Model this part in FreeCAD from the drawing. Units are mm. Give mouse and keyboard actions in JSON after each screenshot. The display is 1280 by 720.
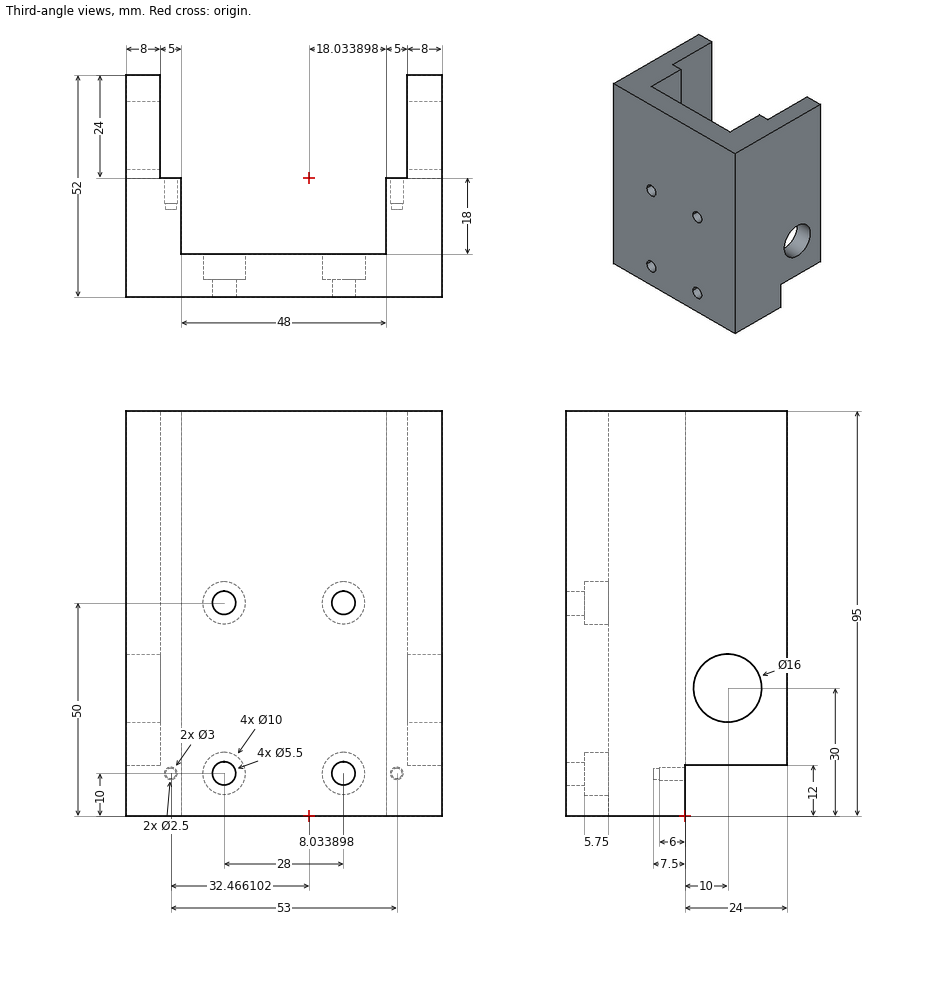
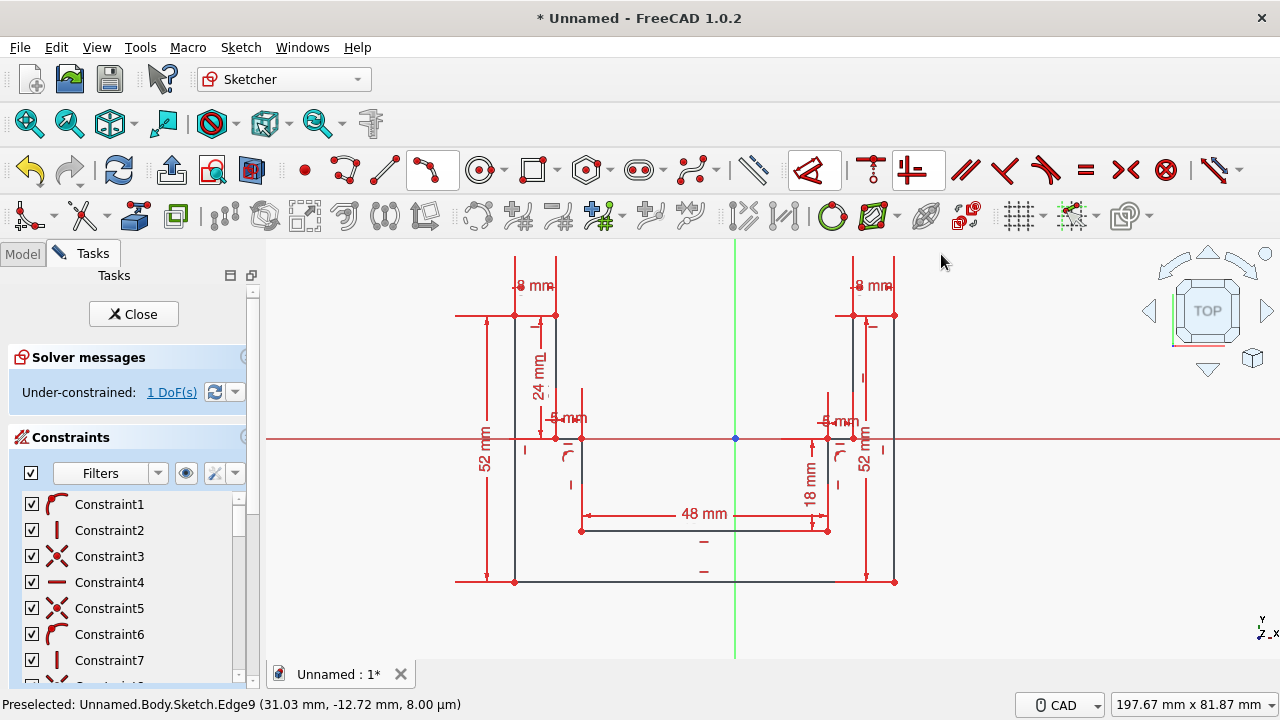
{"action": "left_click", "coordinate": [828, 439]}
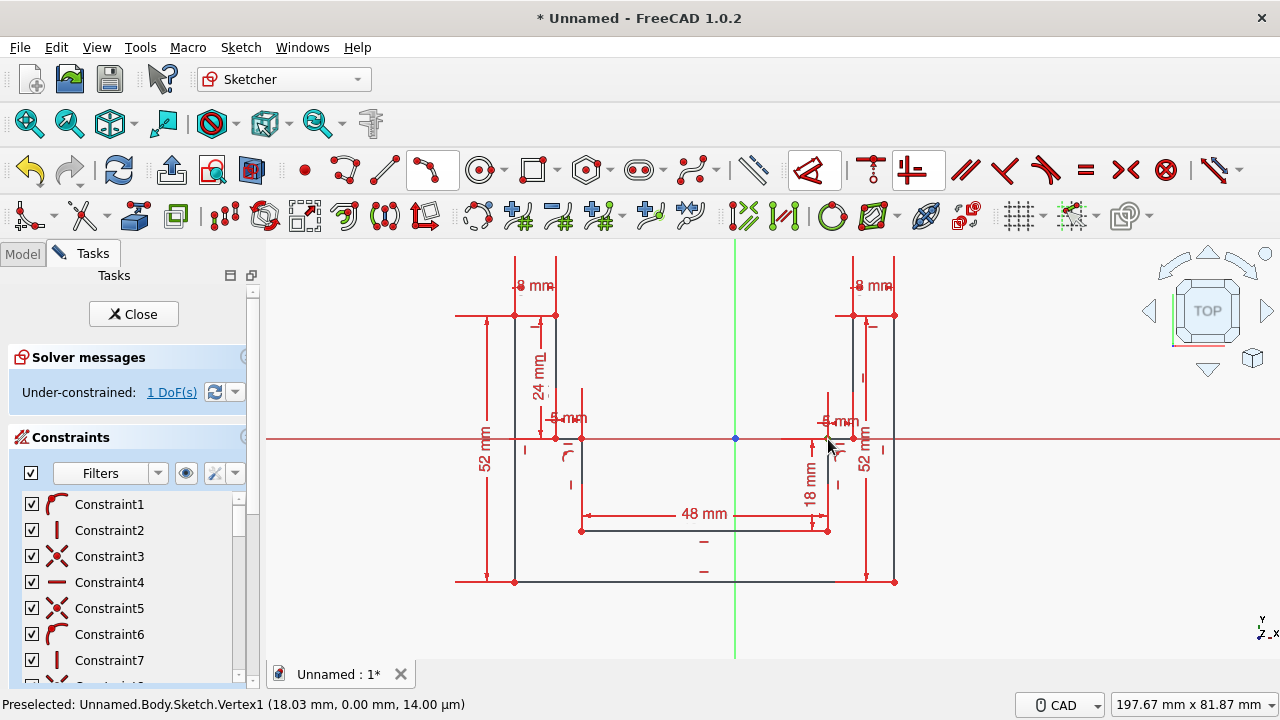
{"action": "key", "text": "l"}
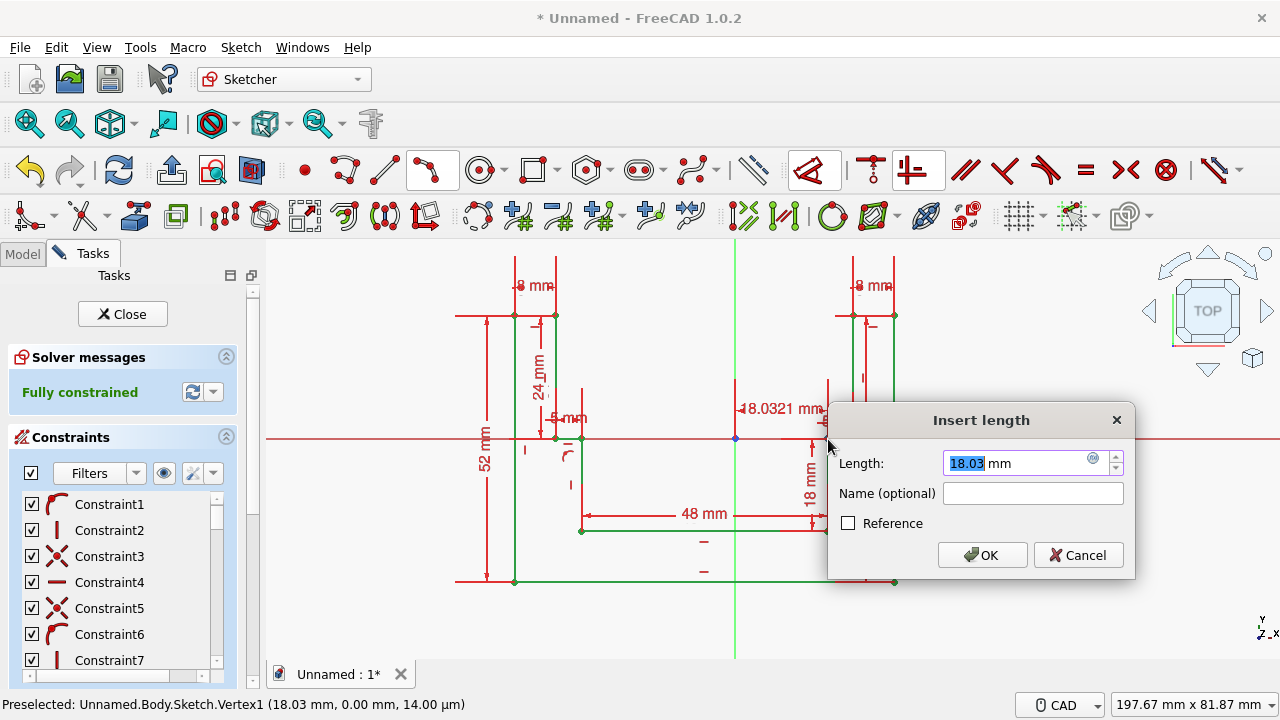
{"action": "type", "text": "18.033898"}
{"action": "key", "text": "Return"}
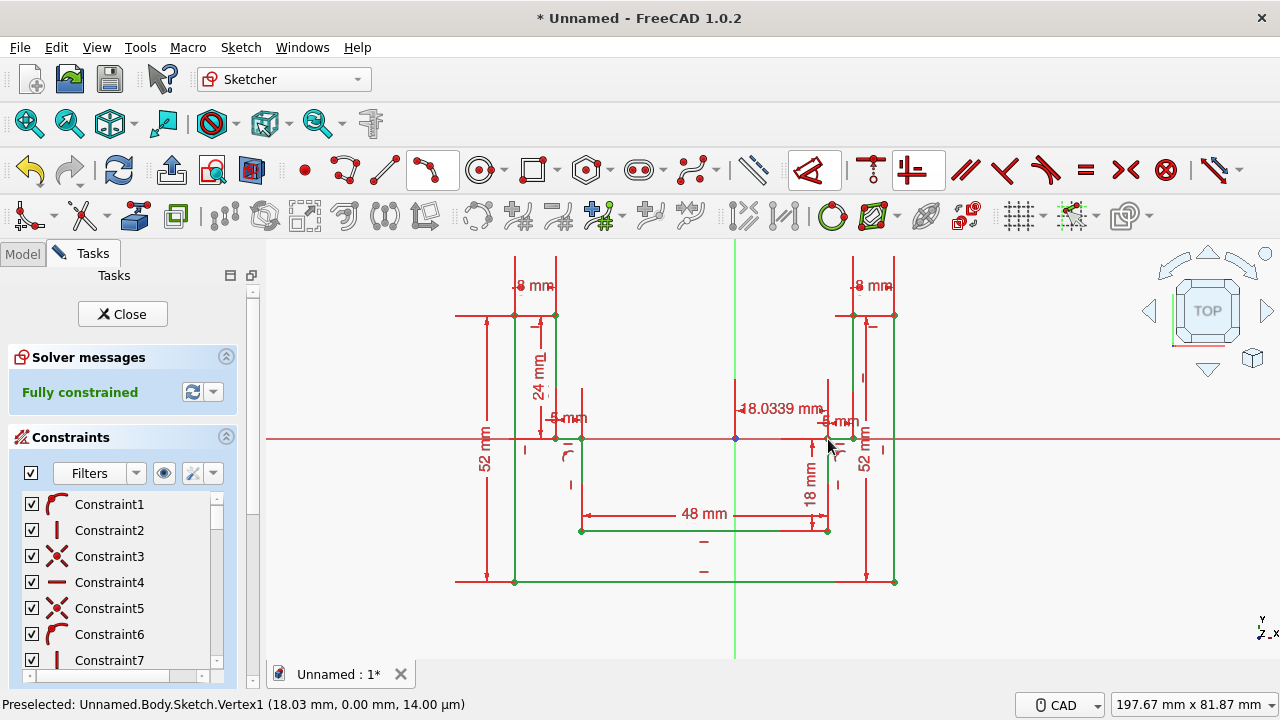
{"action": "left_click", "coordinate": [123, 314]}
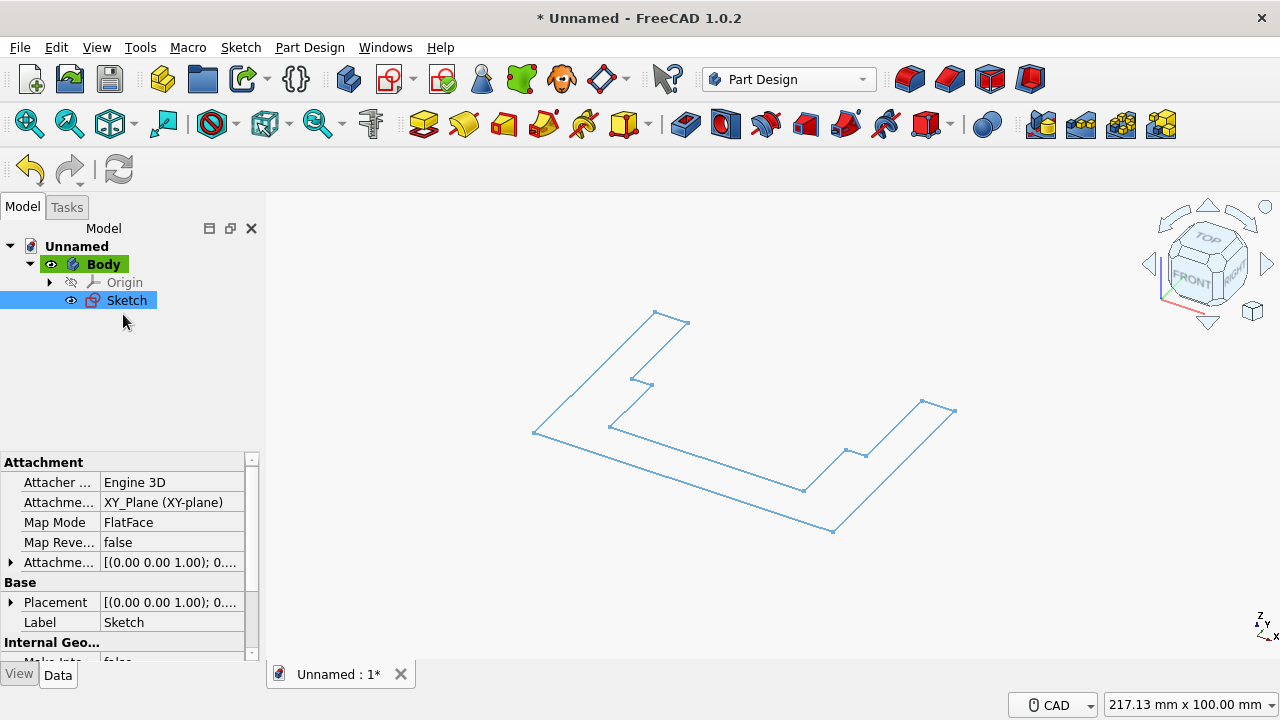
{"action": "left_click", "coordinate": [424, 124]}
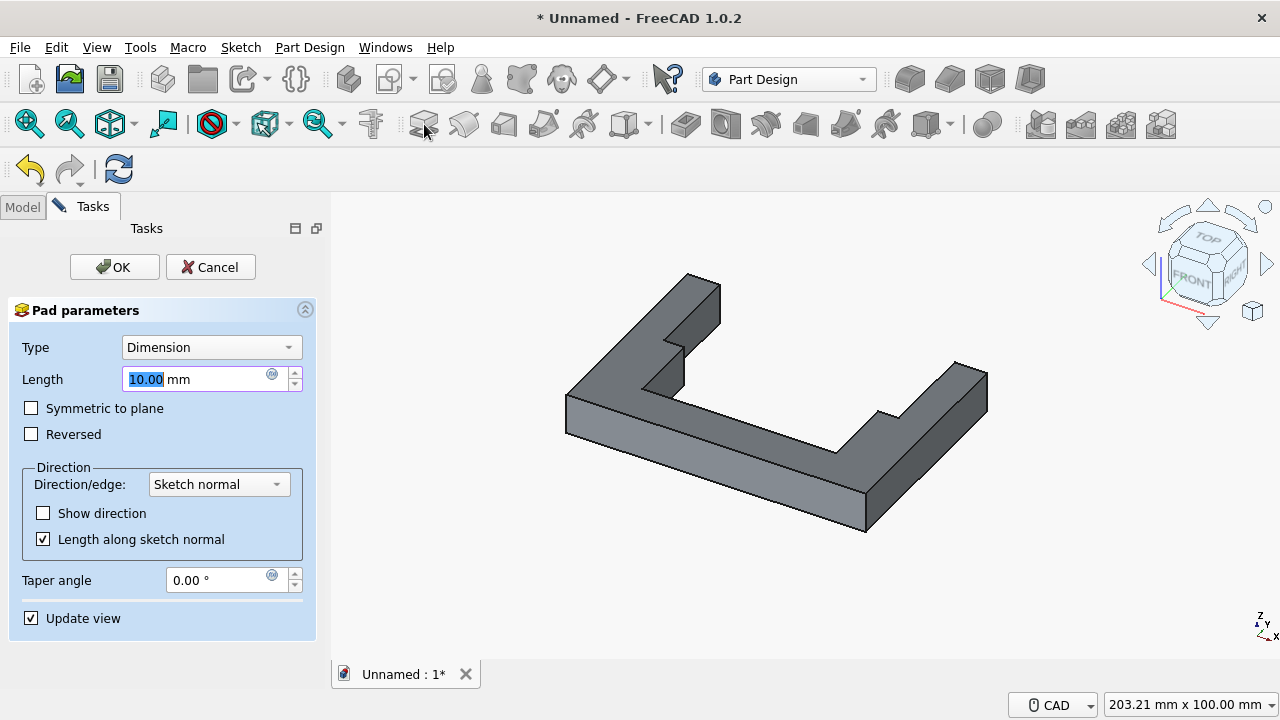
{"action": "type", "text": "95"}
{"action": "key", "text": "Tab"}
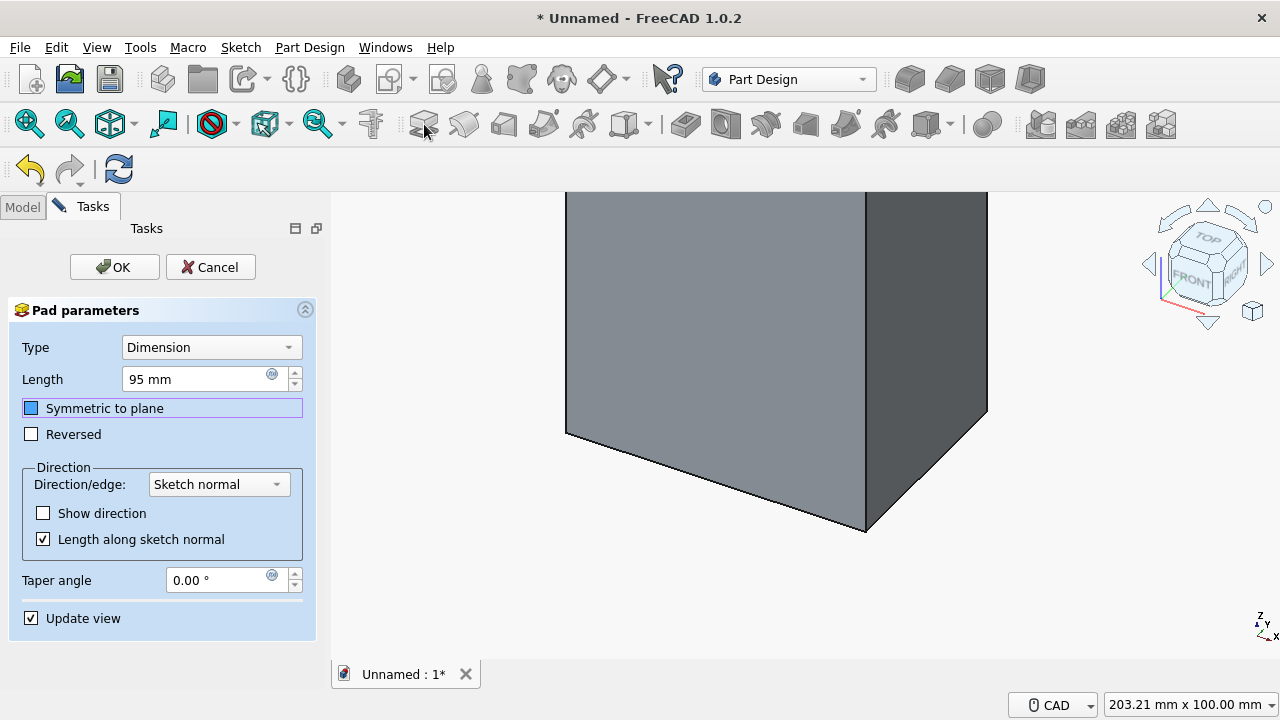
{"action": "left_click", "coordinate": [115, 267]}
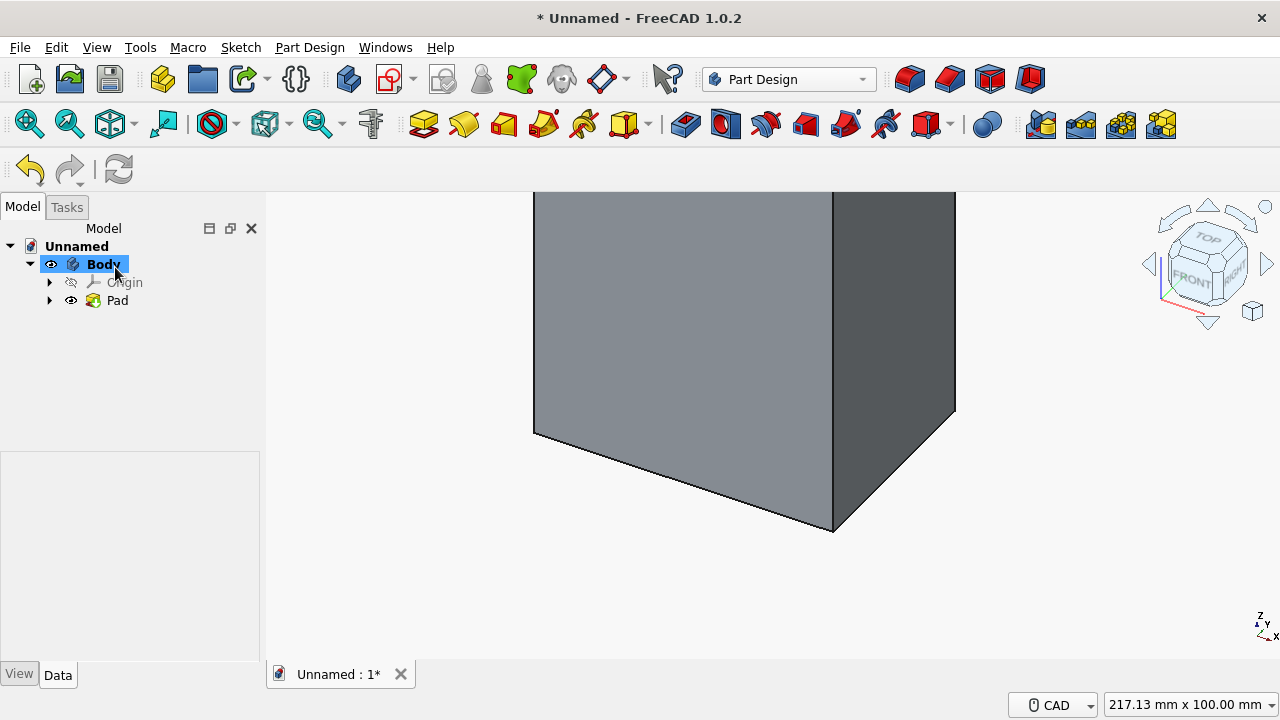
{"action": "left_click", "coordinate": [30, 124]}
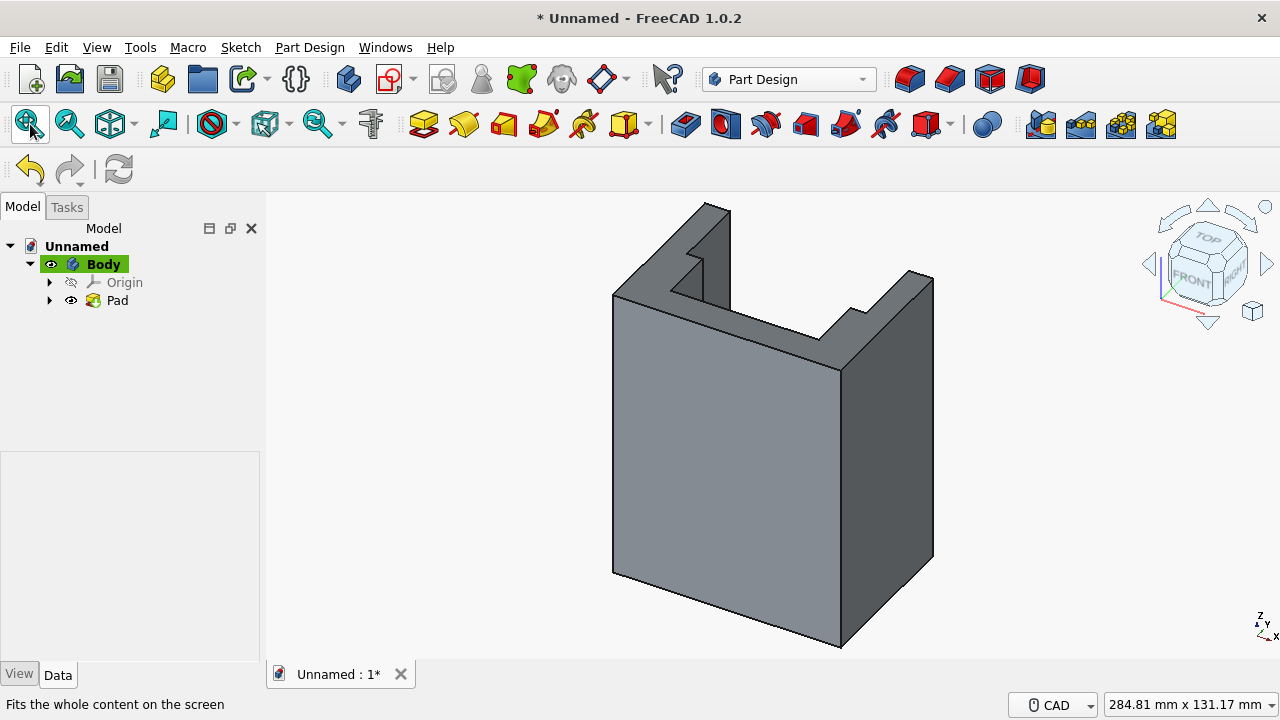
{"action": "key", "text": "4"}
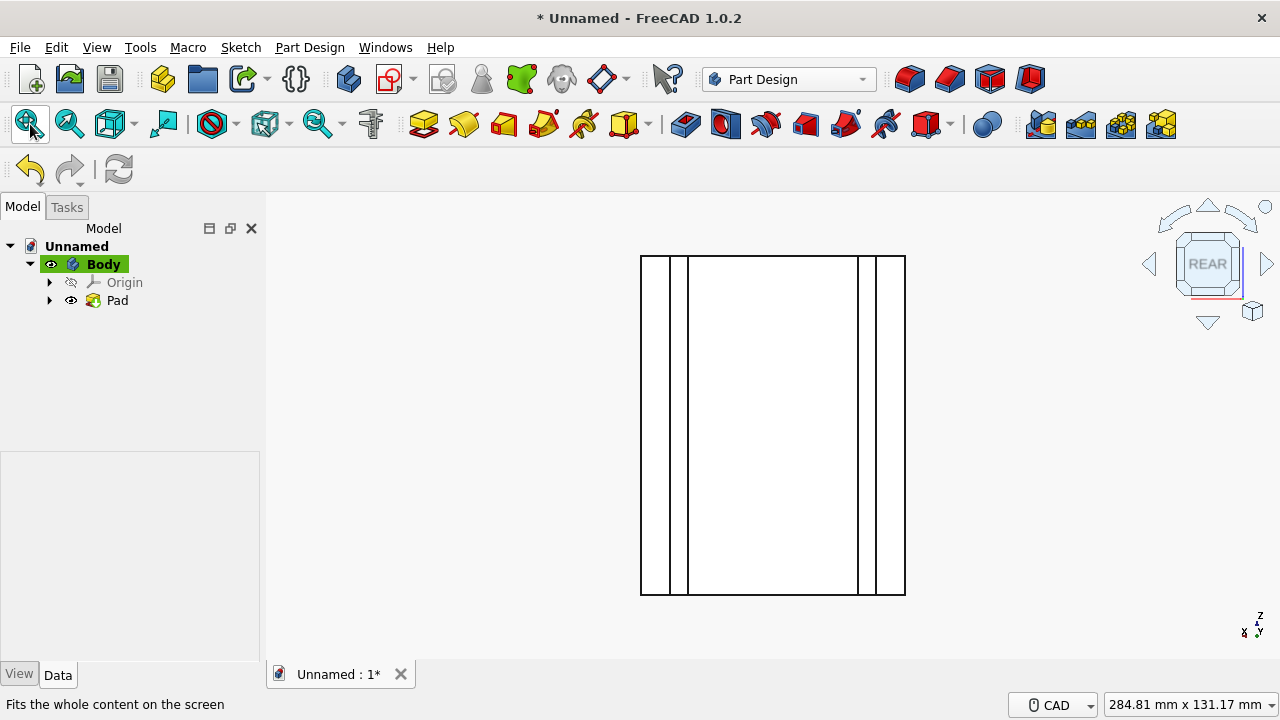
{"action": "left_click", "coordinate": [773, 376]}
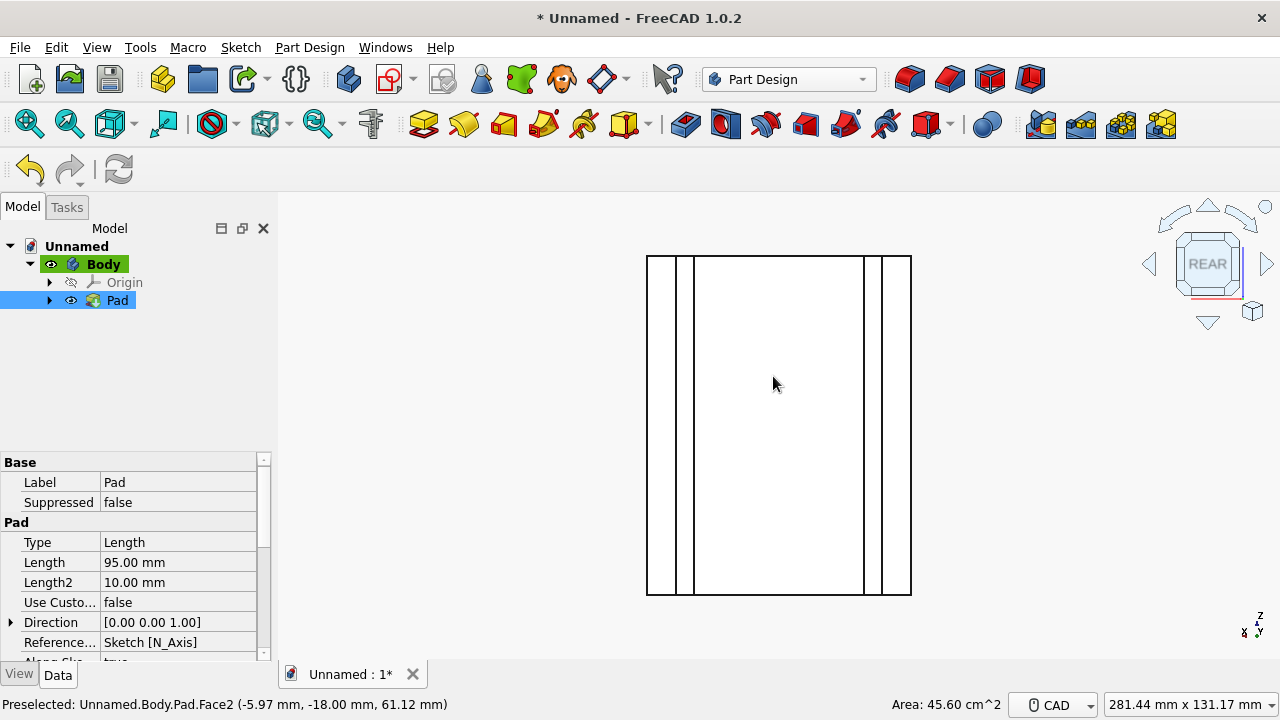
{"action": "left_click", "coordinate": [390, 80]}